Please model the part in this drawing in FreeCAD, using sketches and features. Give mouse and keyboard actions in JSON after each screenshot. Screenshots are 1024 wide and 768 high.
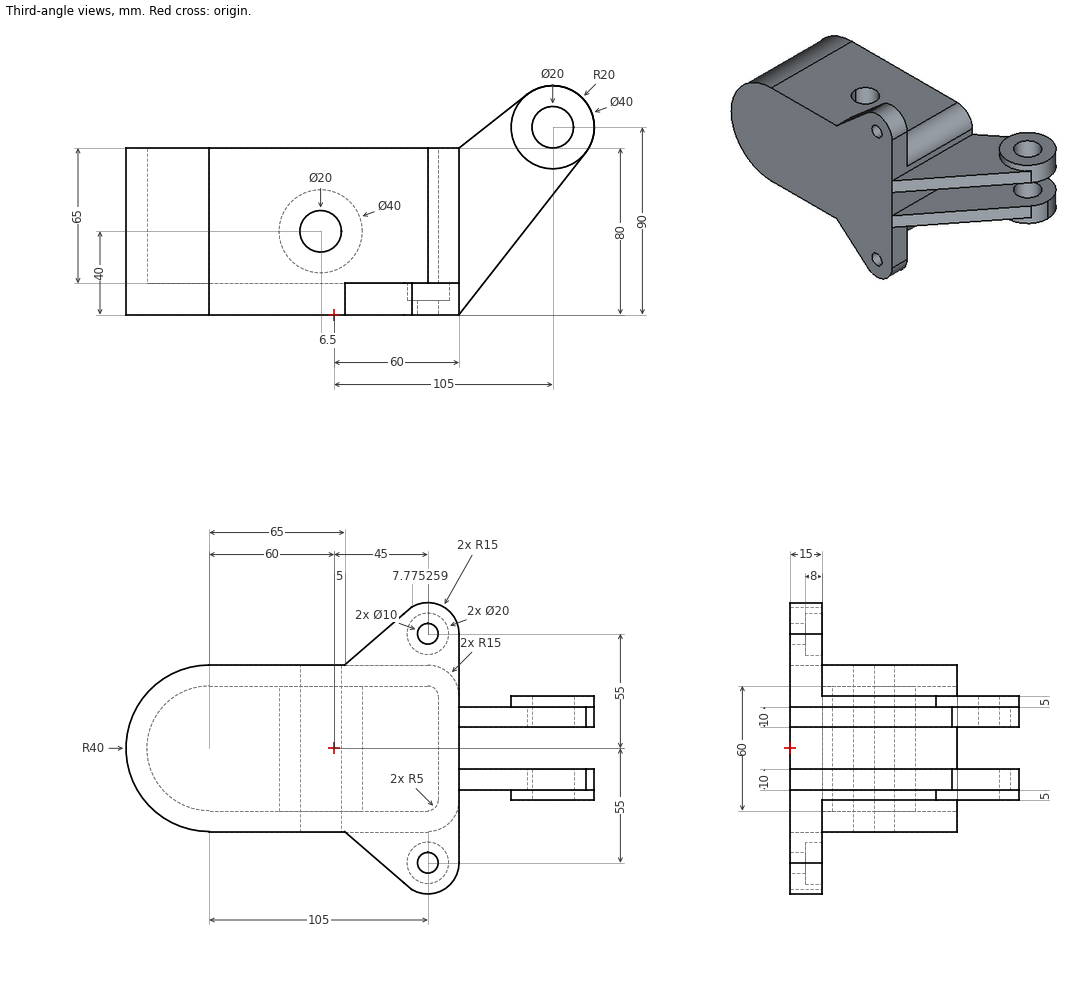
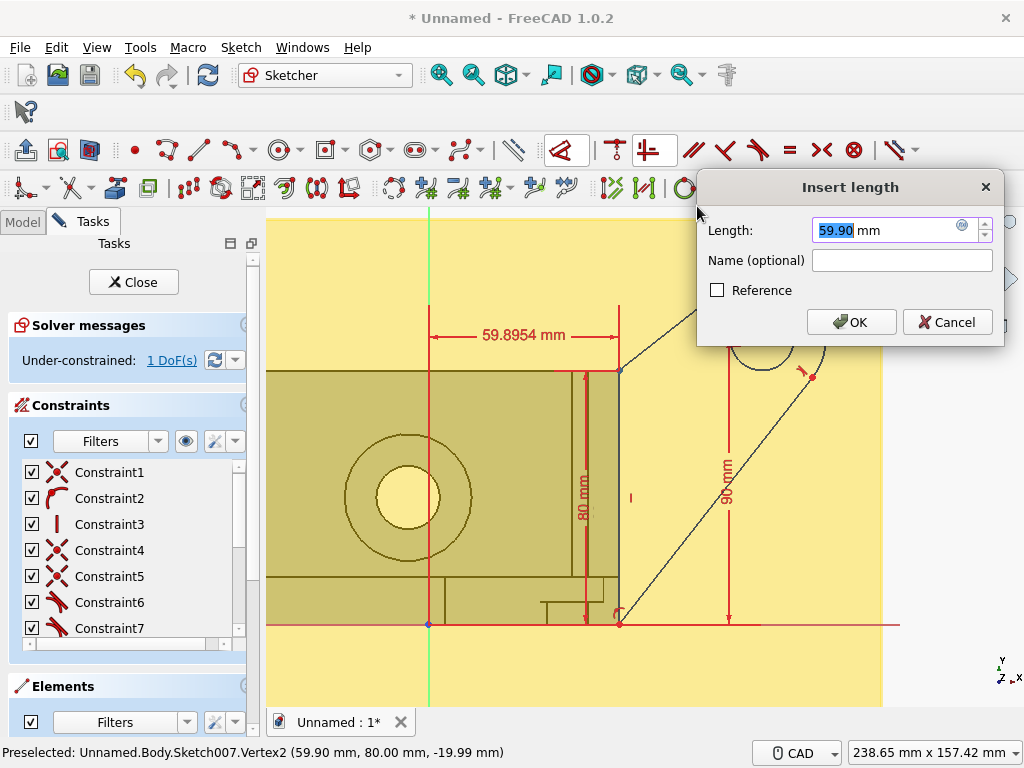
{"action": "type", "text": "60"}
{"action": "key", "text": "Return"}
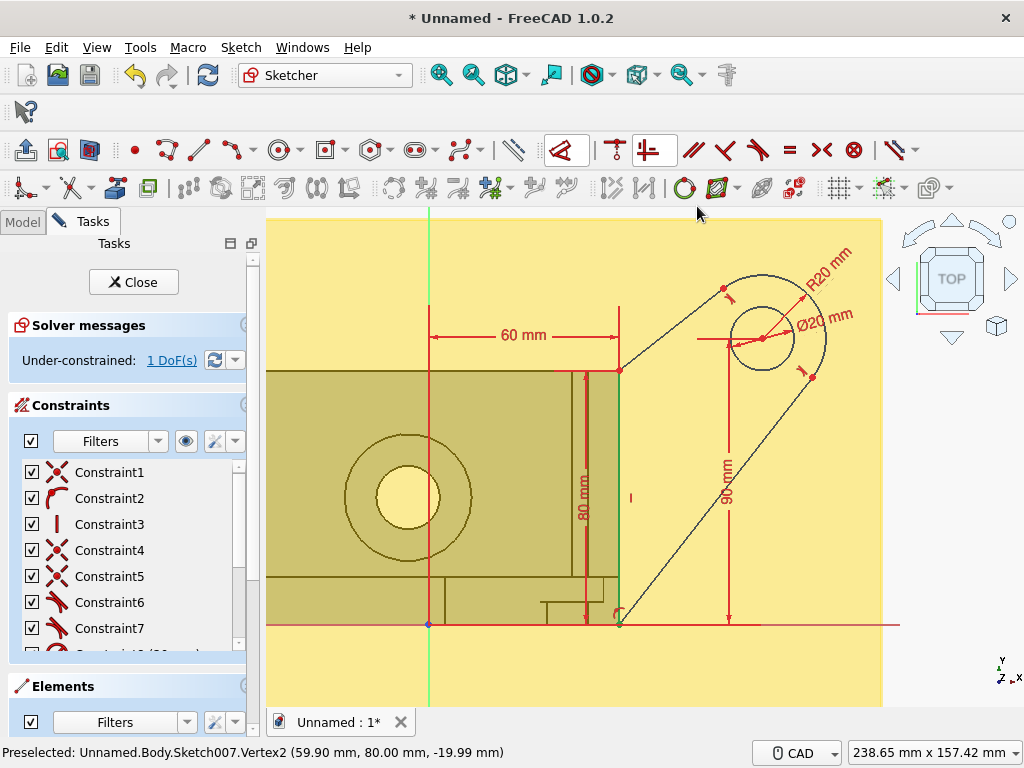
{"action": "left_click", "coordinate": [762, 339]}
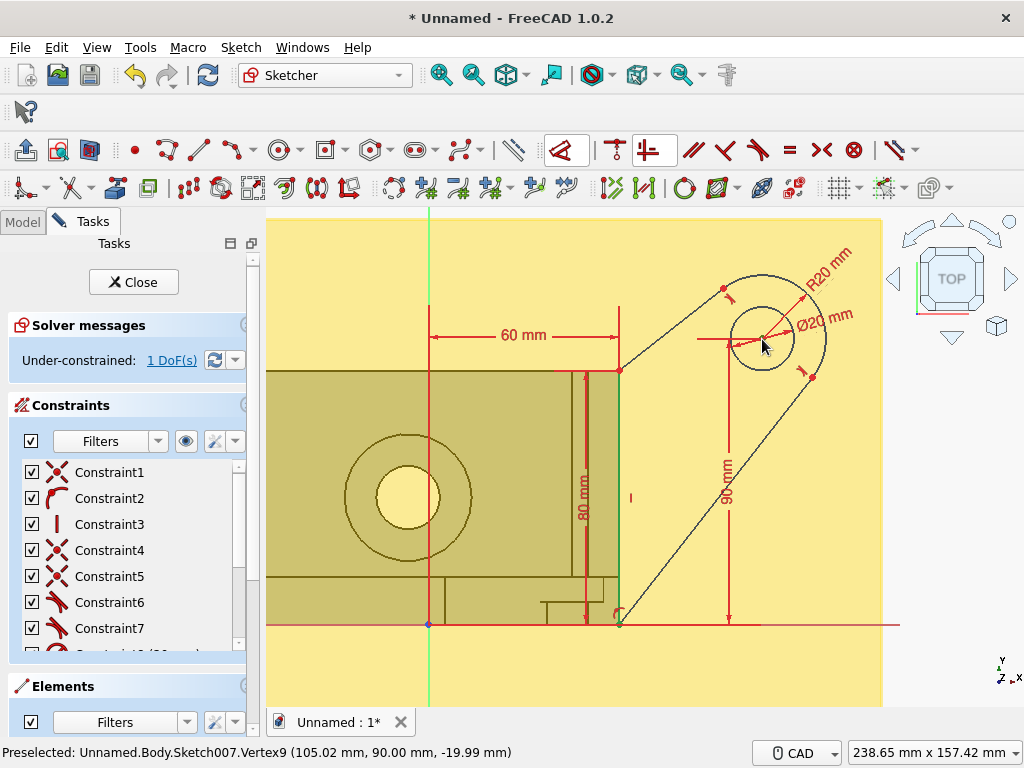
{"action": "key", "text": "l"}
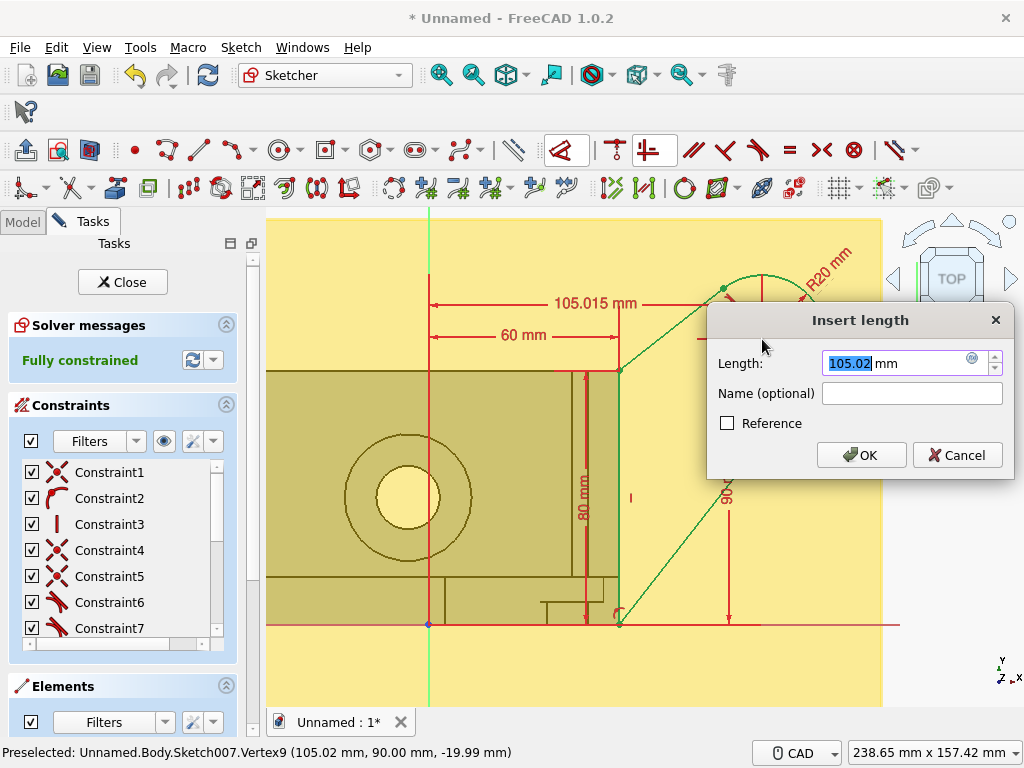
{"action": "type", "text": "105"}
{"action": "key", "text": "Return"}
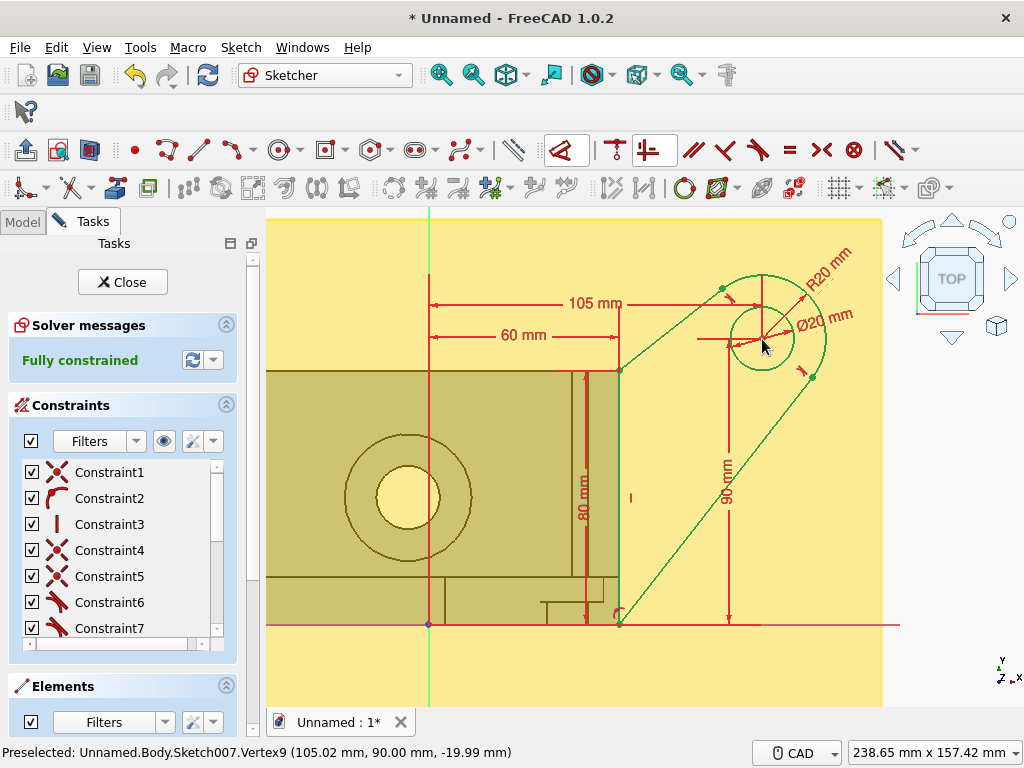
{"action": "left_click", "coordinate": [123, 282]}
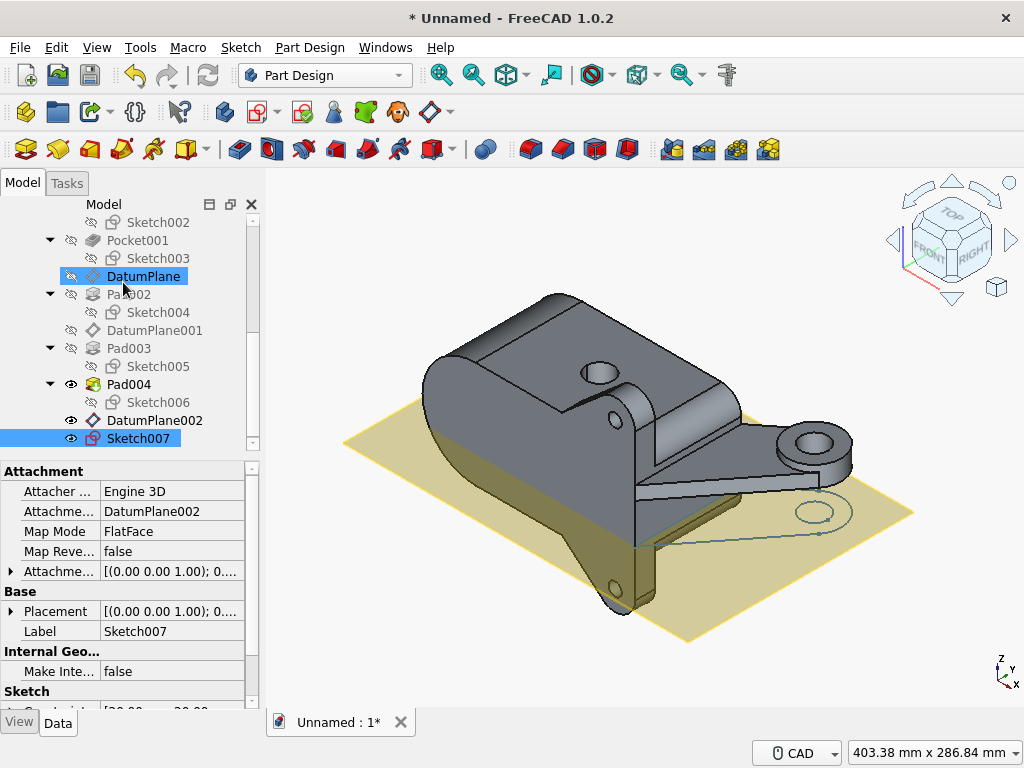
{"action": "left_click", "coordinate": [26, 150]}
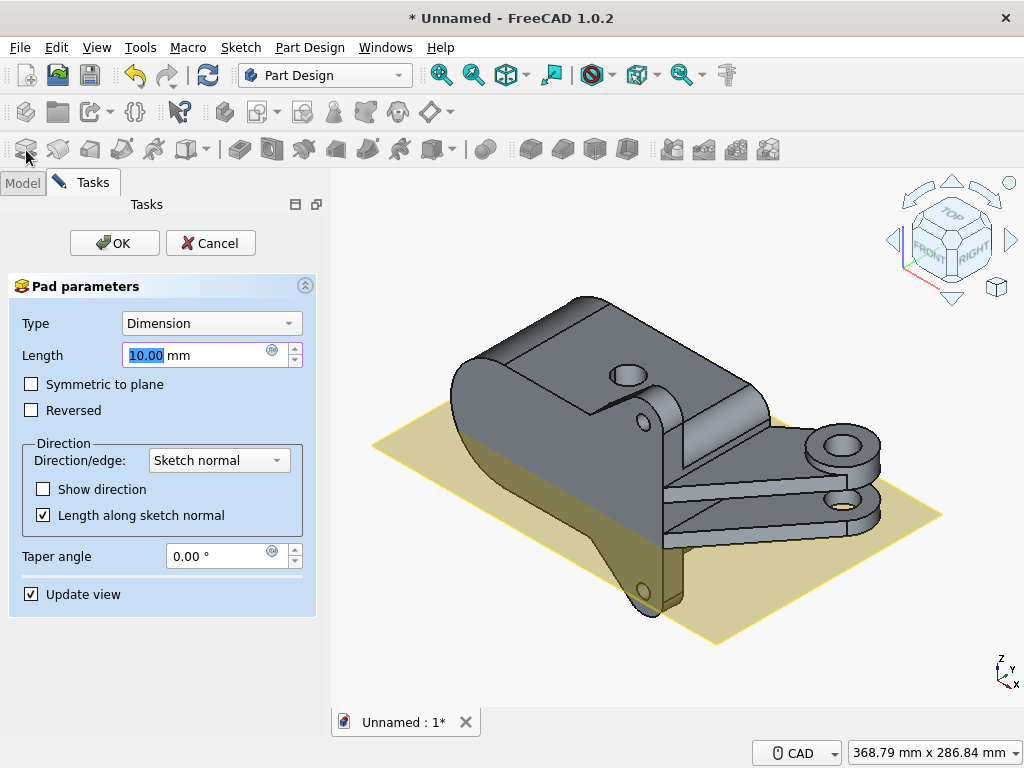
{"action": "type", "text": "10"}
{"action": "key", "text": "Tab"}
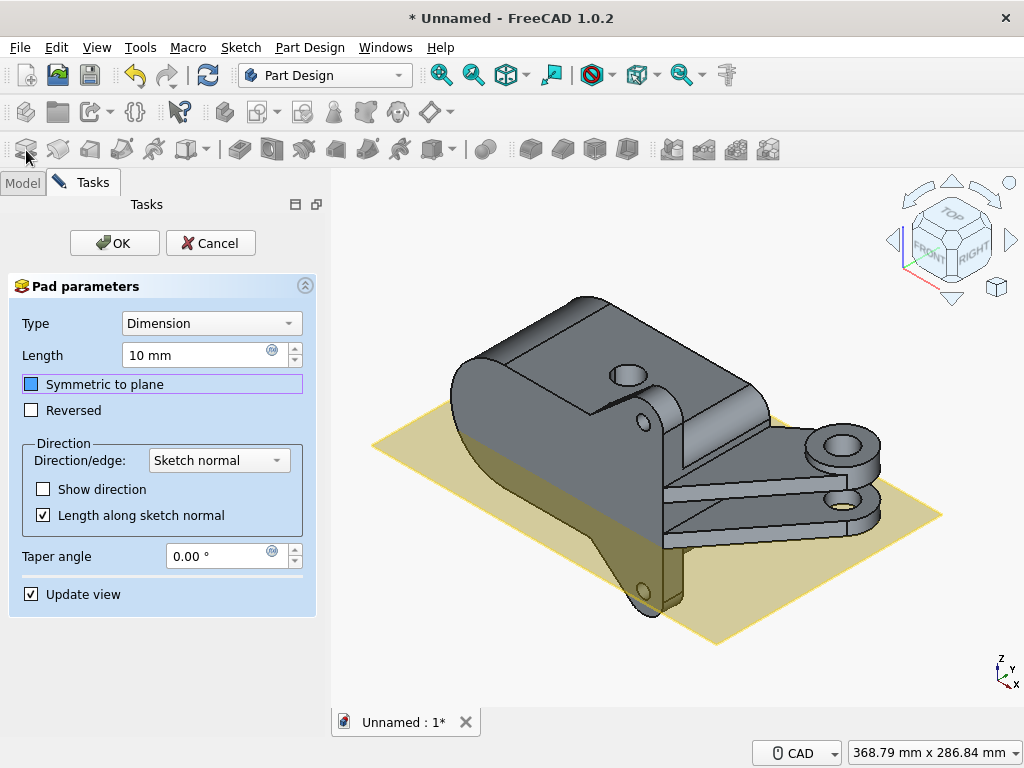
{"action": "left_click", "coordinate": [115, 243]}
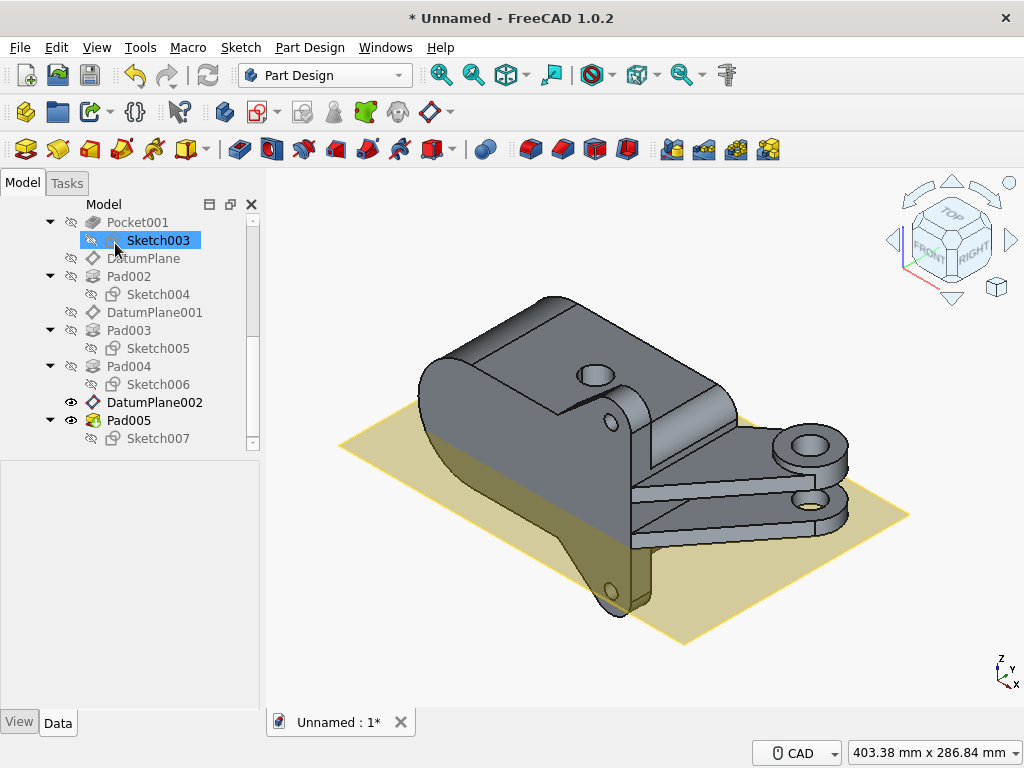
{"action": "left_click", "coordinate": [116, 402]}
{"action": "key", "text": "space"}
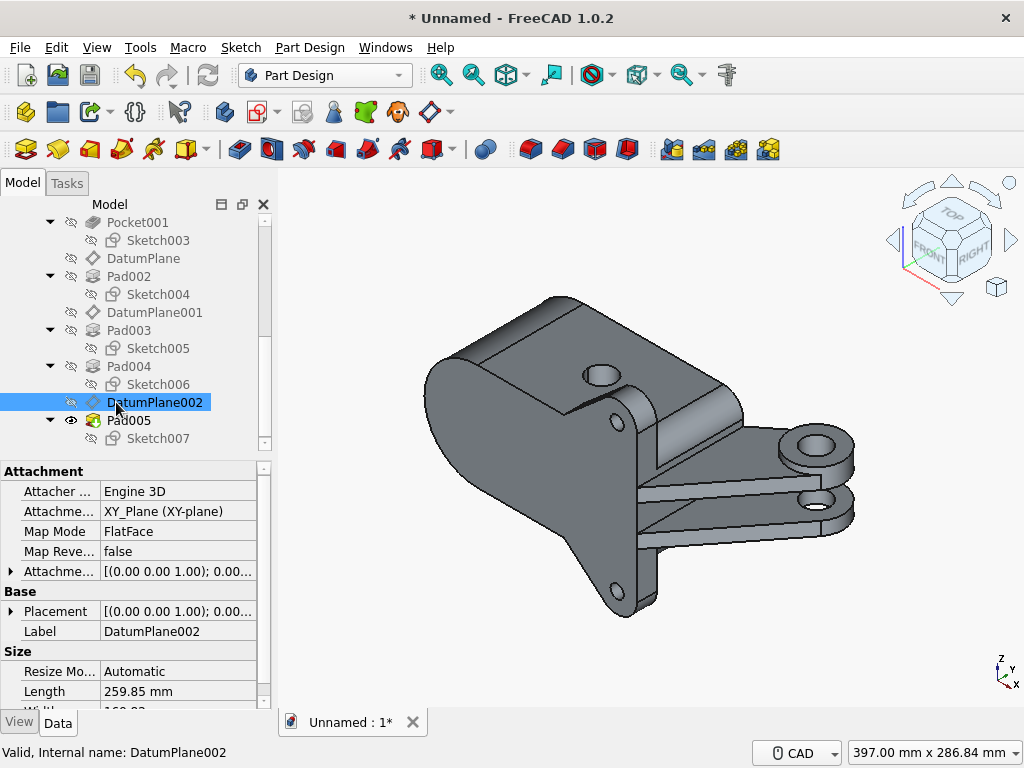
{"action": "scroll", "coordinate": [140, 326], "scroll_direction": "down", "scroll_amount": 3}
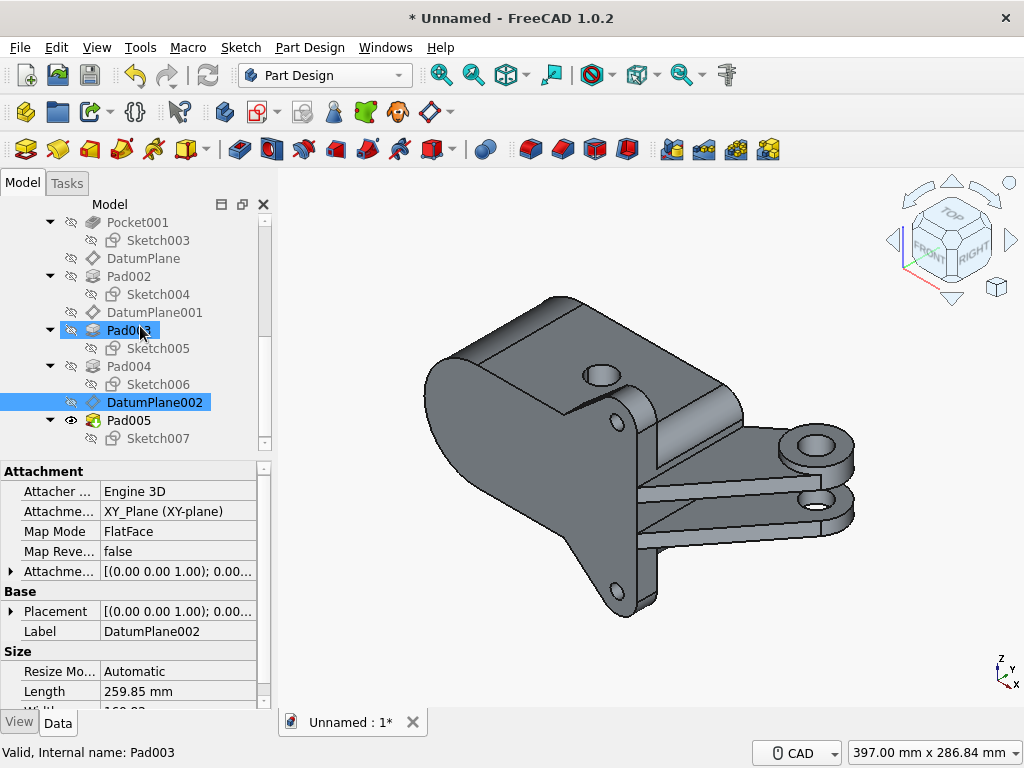
{"action": "scroll", "coordinate": [140, 326], "scroll_direction": "up", "scroll_amount": 15}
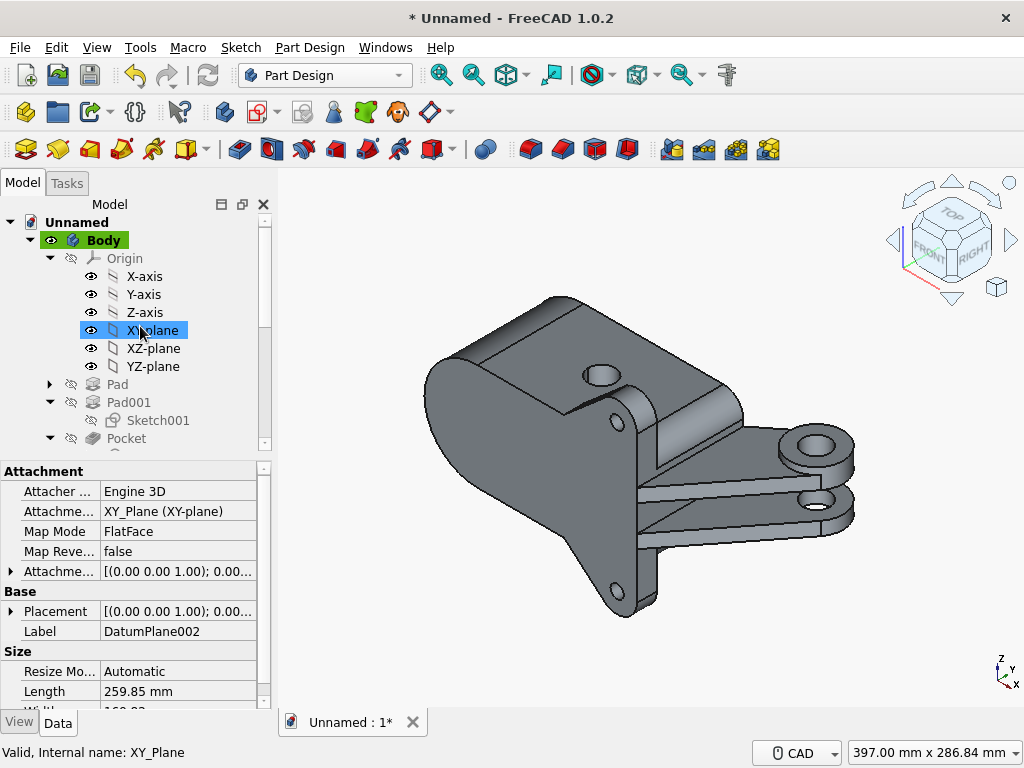
{"action": "left_click", "coordinate": [136, 330]}